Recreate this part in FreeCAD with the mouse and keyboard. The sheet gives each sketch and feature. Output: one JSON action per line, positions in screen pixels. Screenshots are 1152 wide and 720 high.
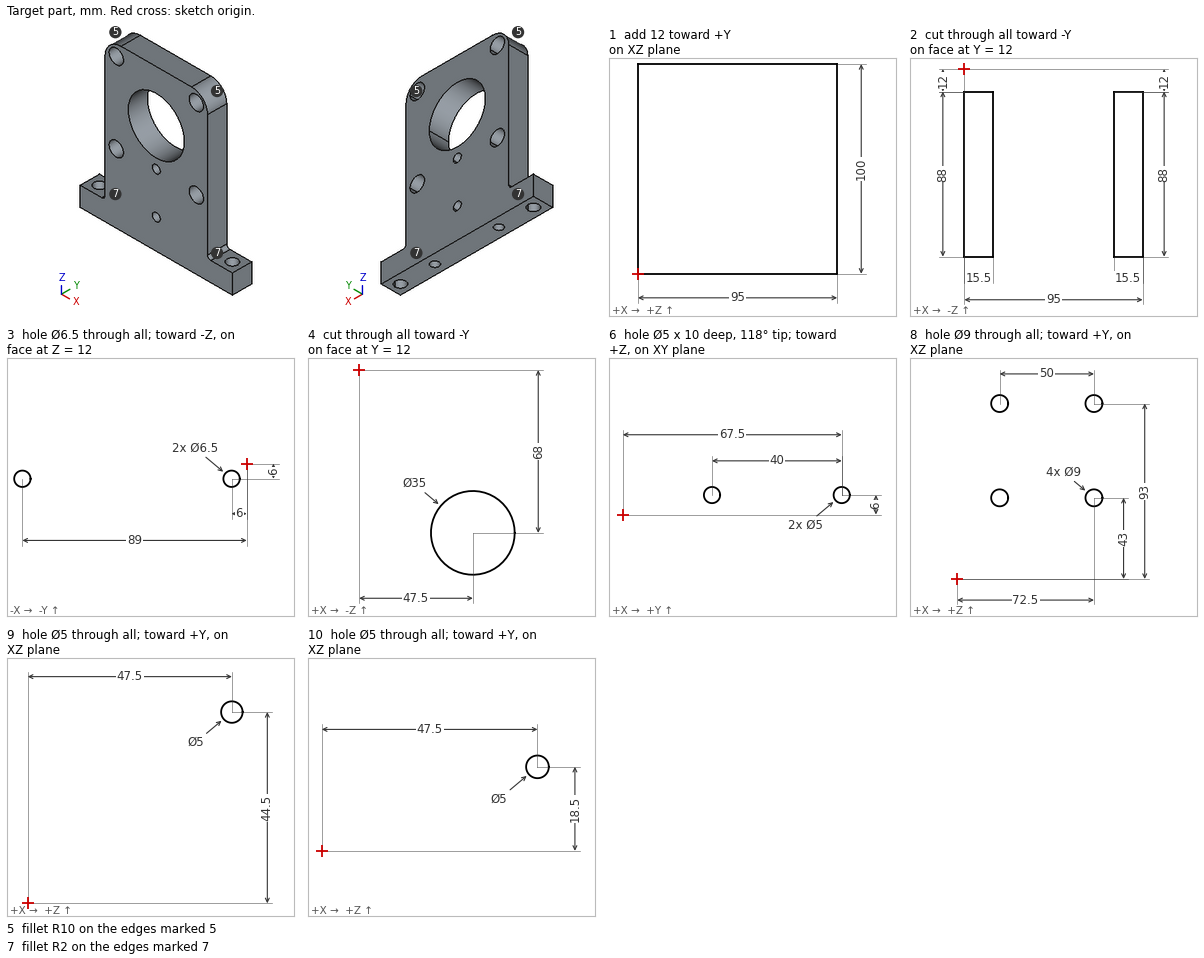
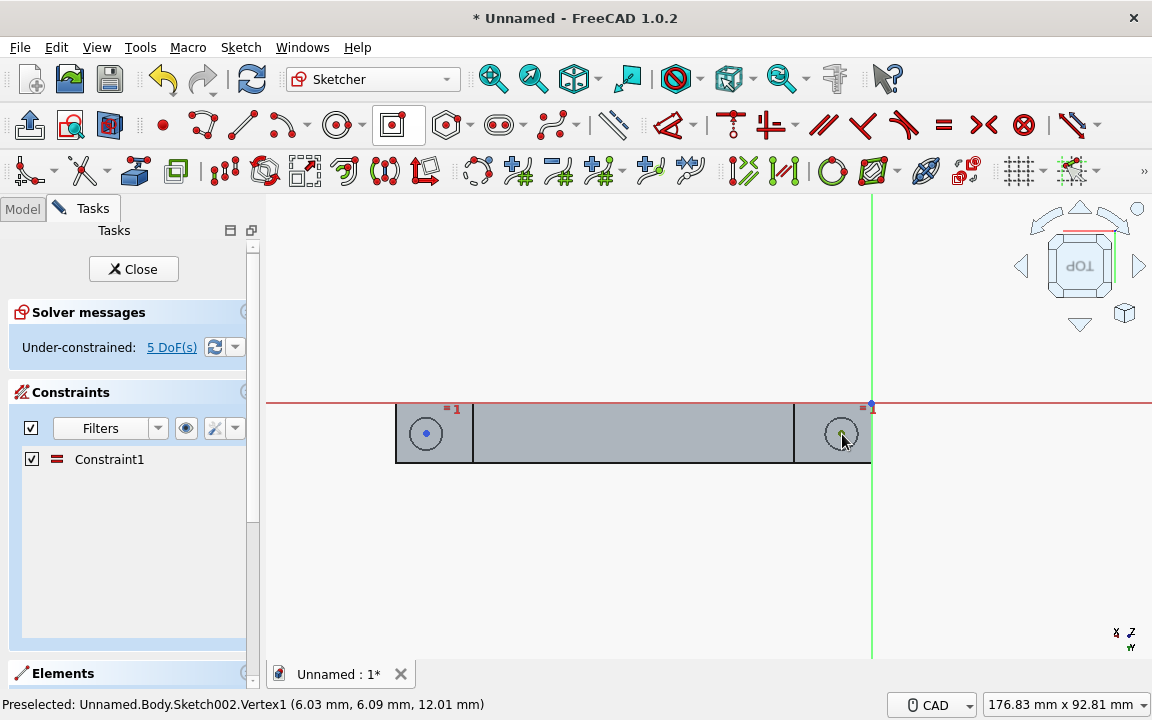
{"action": "left_click", "coordinate": [426, 434]}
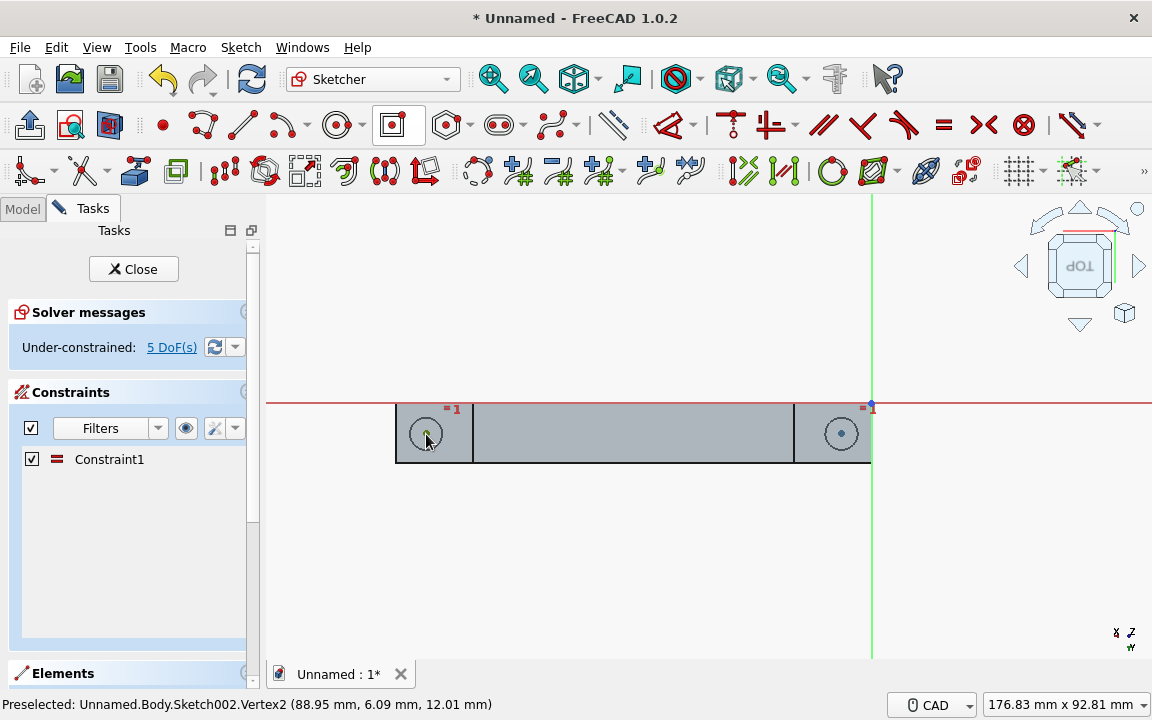
{"action": "key", "text": "h"}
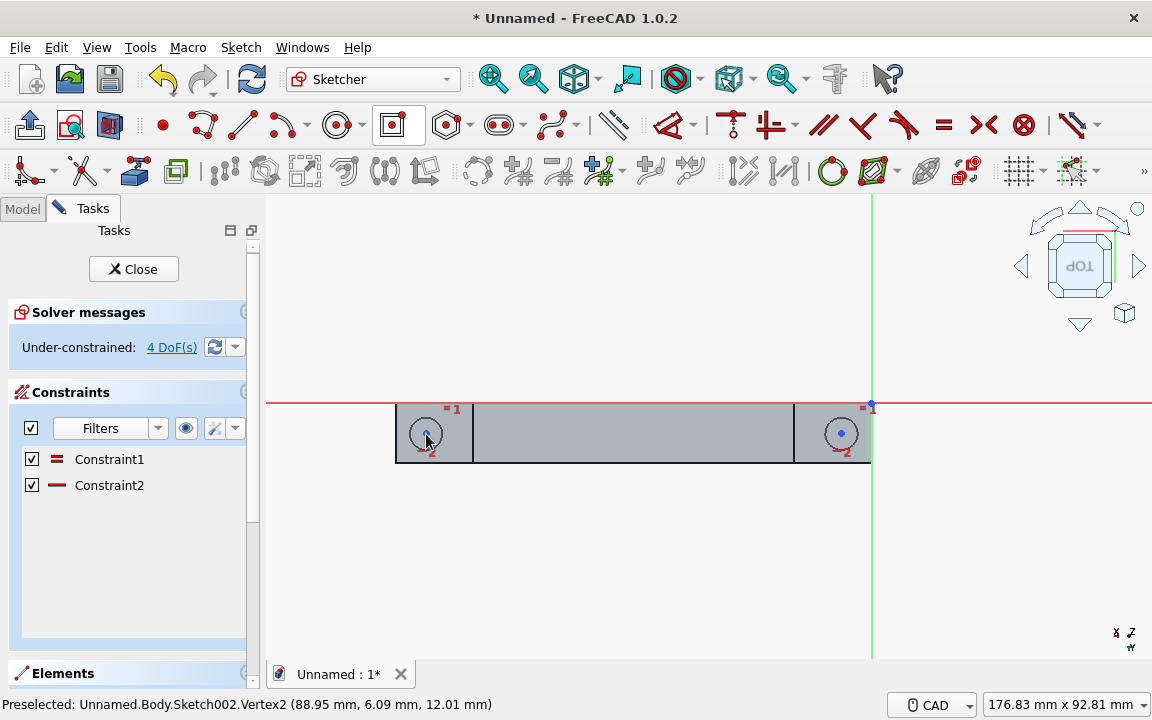
{"action": "left_click", "coordinate": [668, 126]}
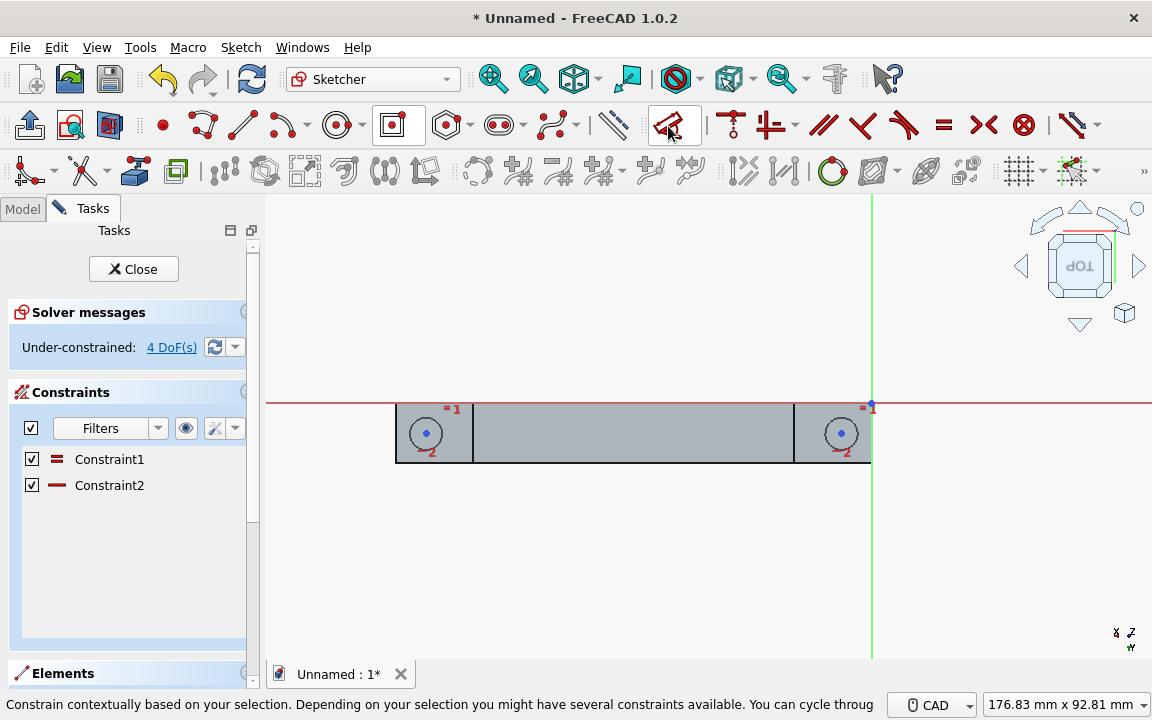
{"action": "left_click", "coordinate": [853, 422]}
{"action": "left_click", "coordinate": [888, 419]}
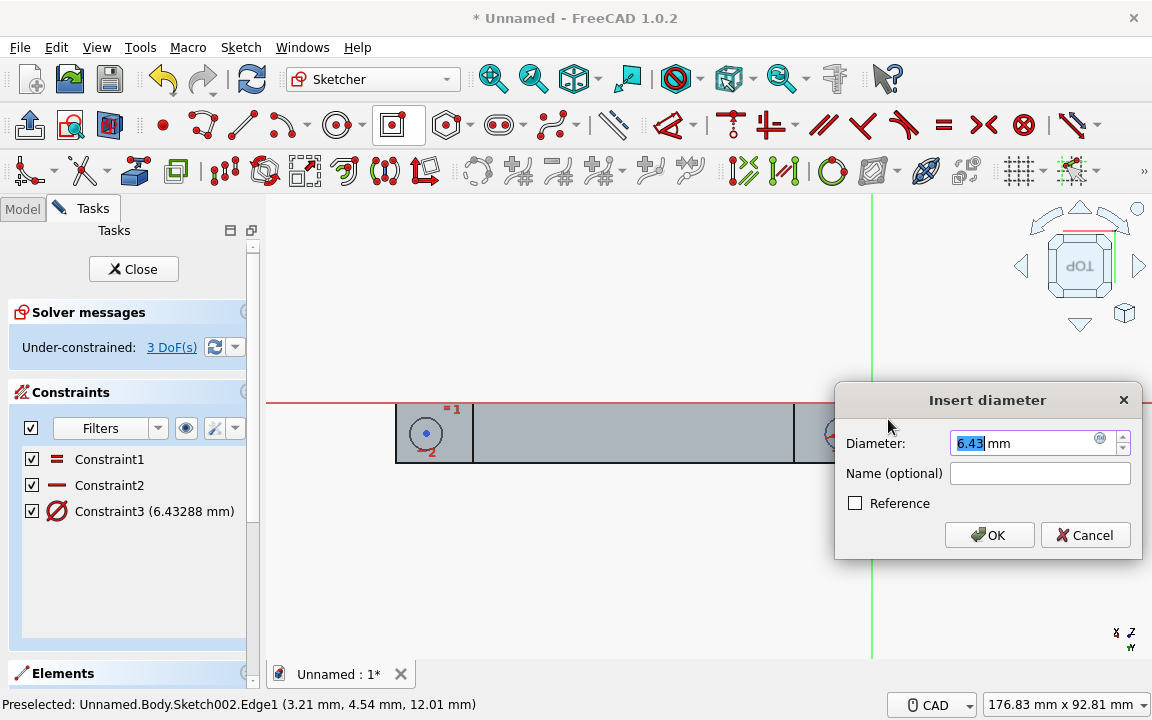
{"action": "type", "text": "6.5"}
{"action": "key", "text": "Return"}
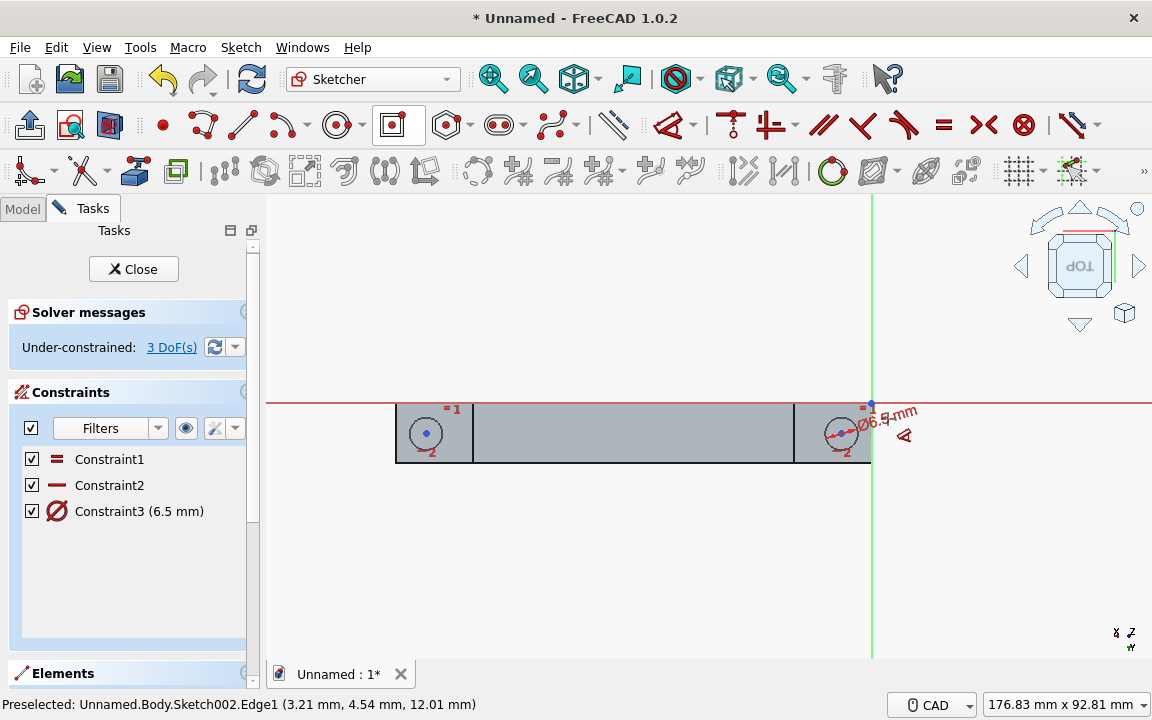
{"action": "scroll", "coordinate": [842, 434], "scroll_direction": "up", "scroll_amount": 2}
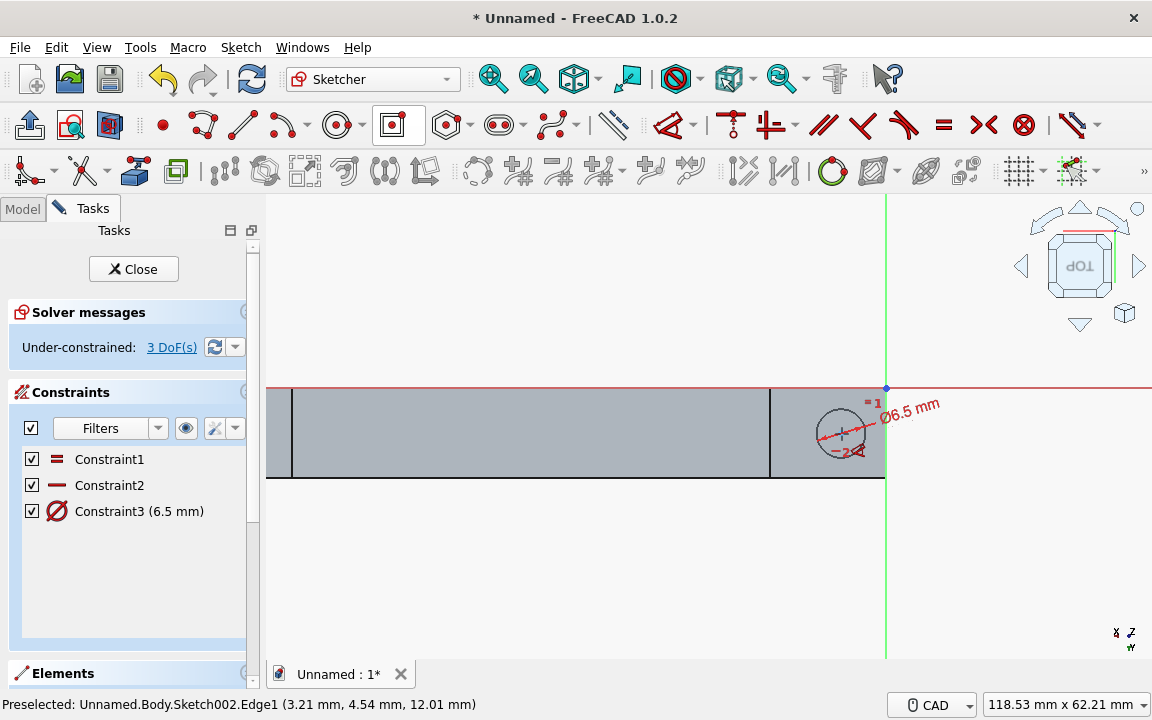
{"action": "left_click", "coordinate": [841, 434]}
{"action": "left_click", "coordinate": [864, 354]}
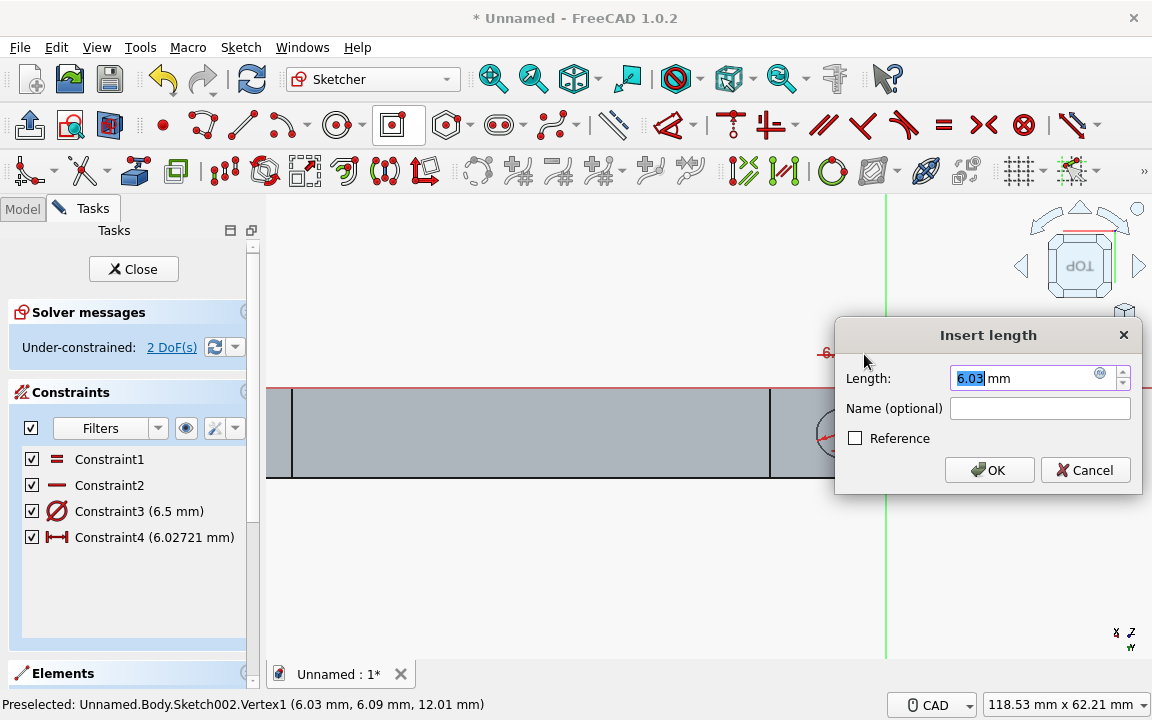
{"action": "type", "text": "6"}
{"action": "key", "text": "Return"}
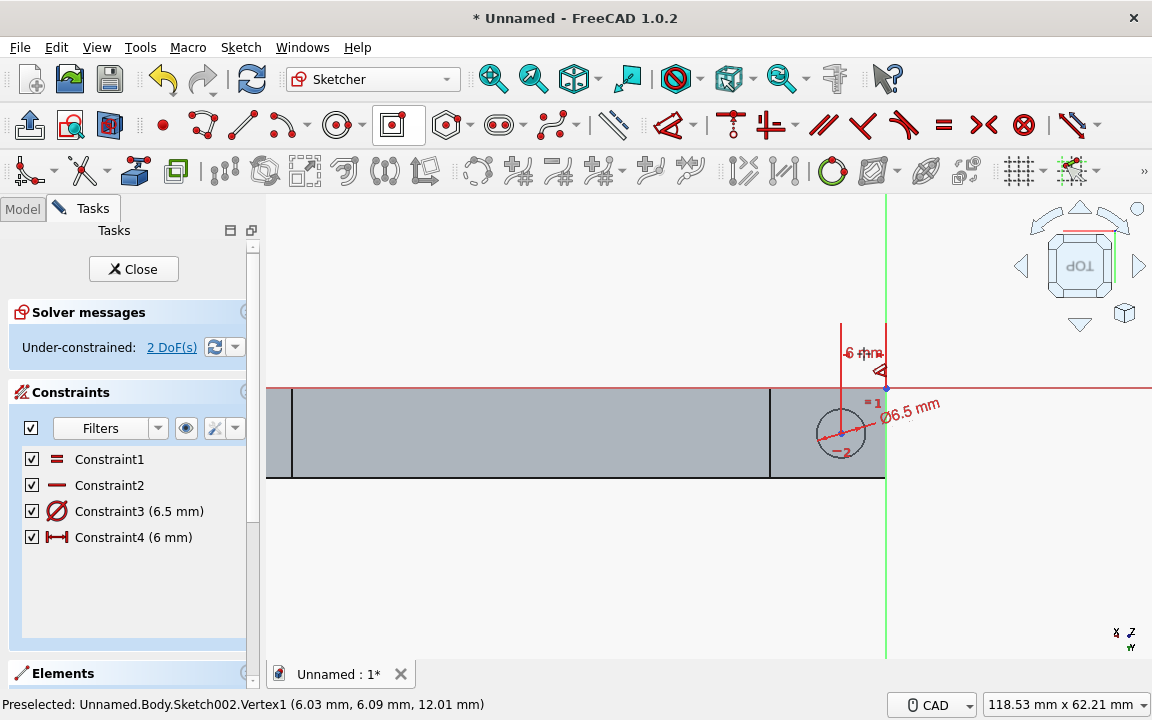
{"action": "left_click", "coordinate": [841, 434]}
{"action": "left_click", "coordinate": [807, 411]}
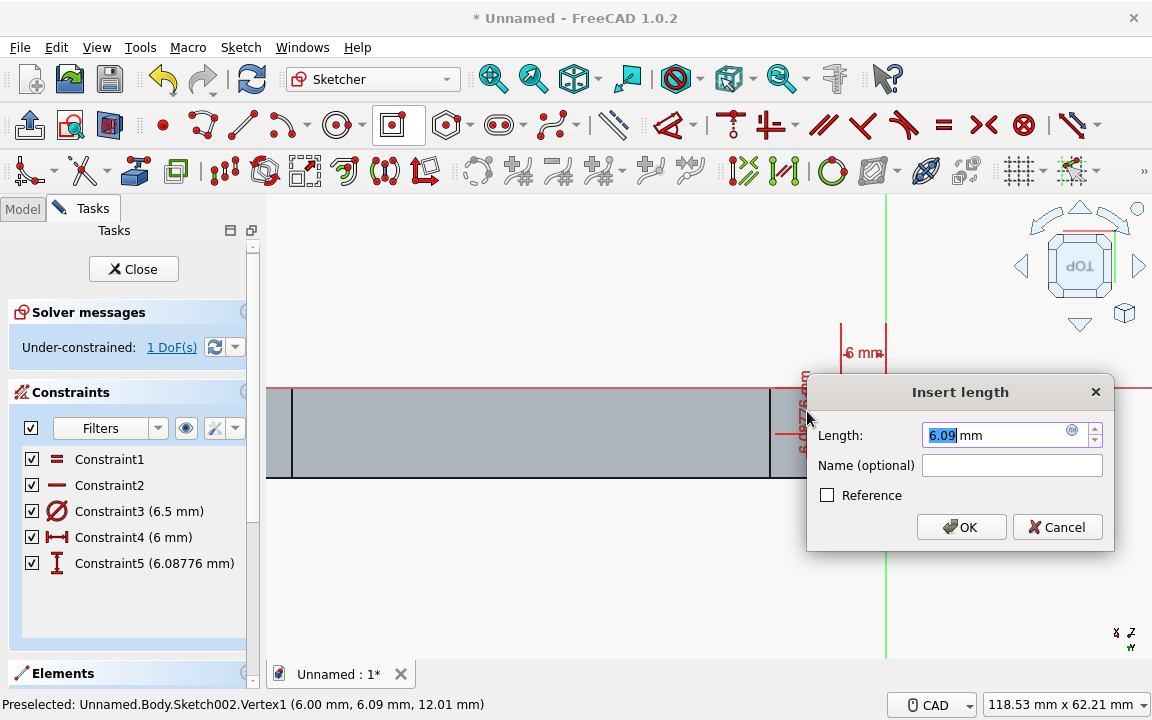
{"action": "type", "text": "6"}
{"action": "key", "text": "Return"}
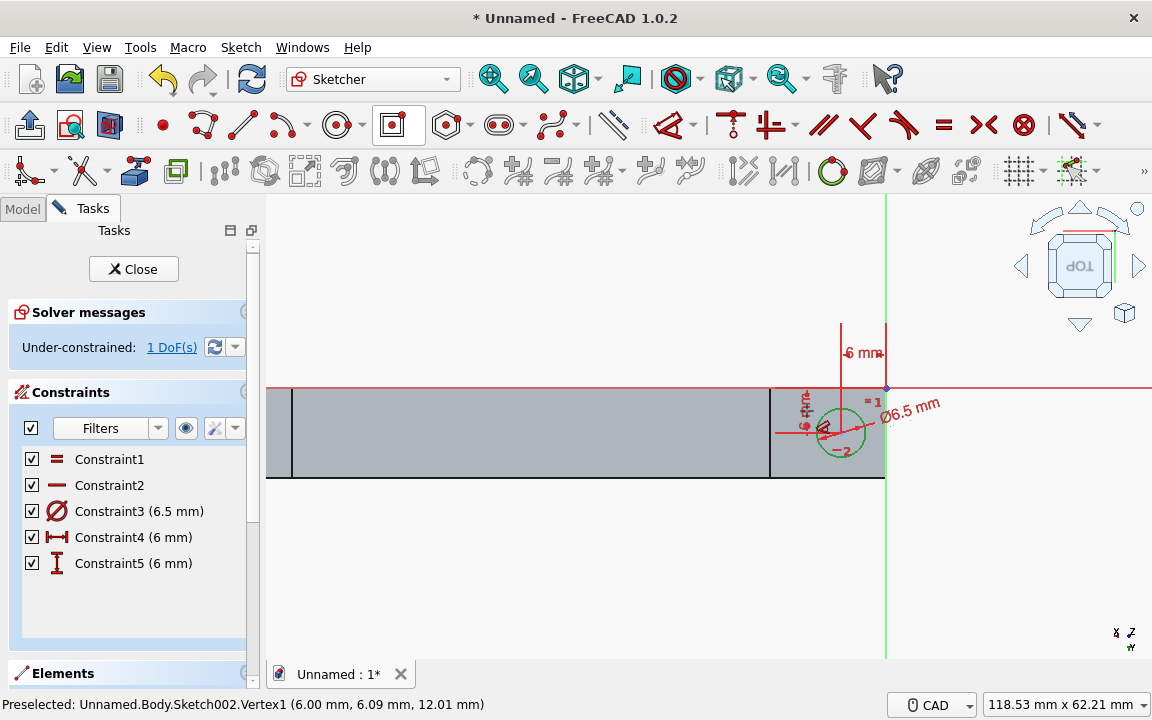
{"action": "scroll", "coordinate": [842, 434], "scroll_direction": "down", "scroll_amount": 2}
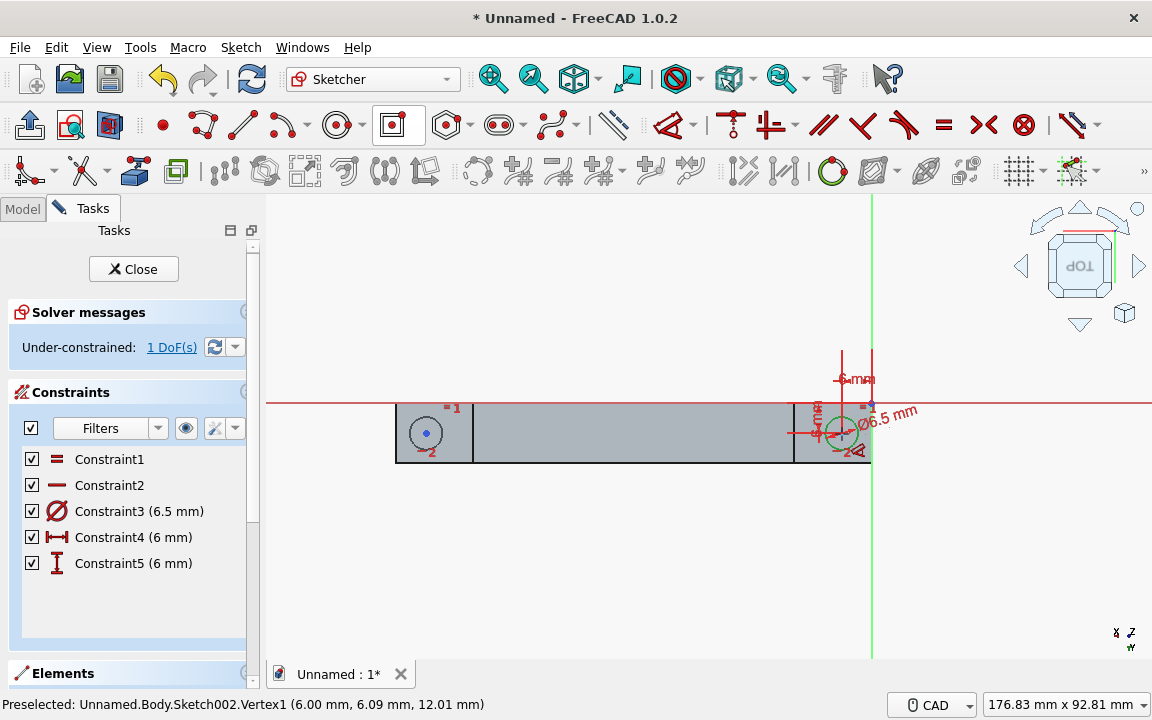
{"action": "left_click", "coordinate": [426, 433]}
{"action": "left_click", "coordinate": [649, 369]}